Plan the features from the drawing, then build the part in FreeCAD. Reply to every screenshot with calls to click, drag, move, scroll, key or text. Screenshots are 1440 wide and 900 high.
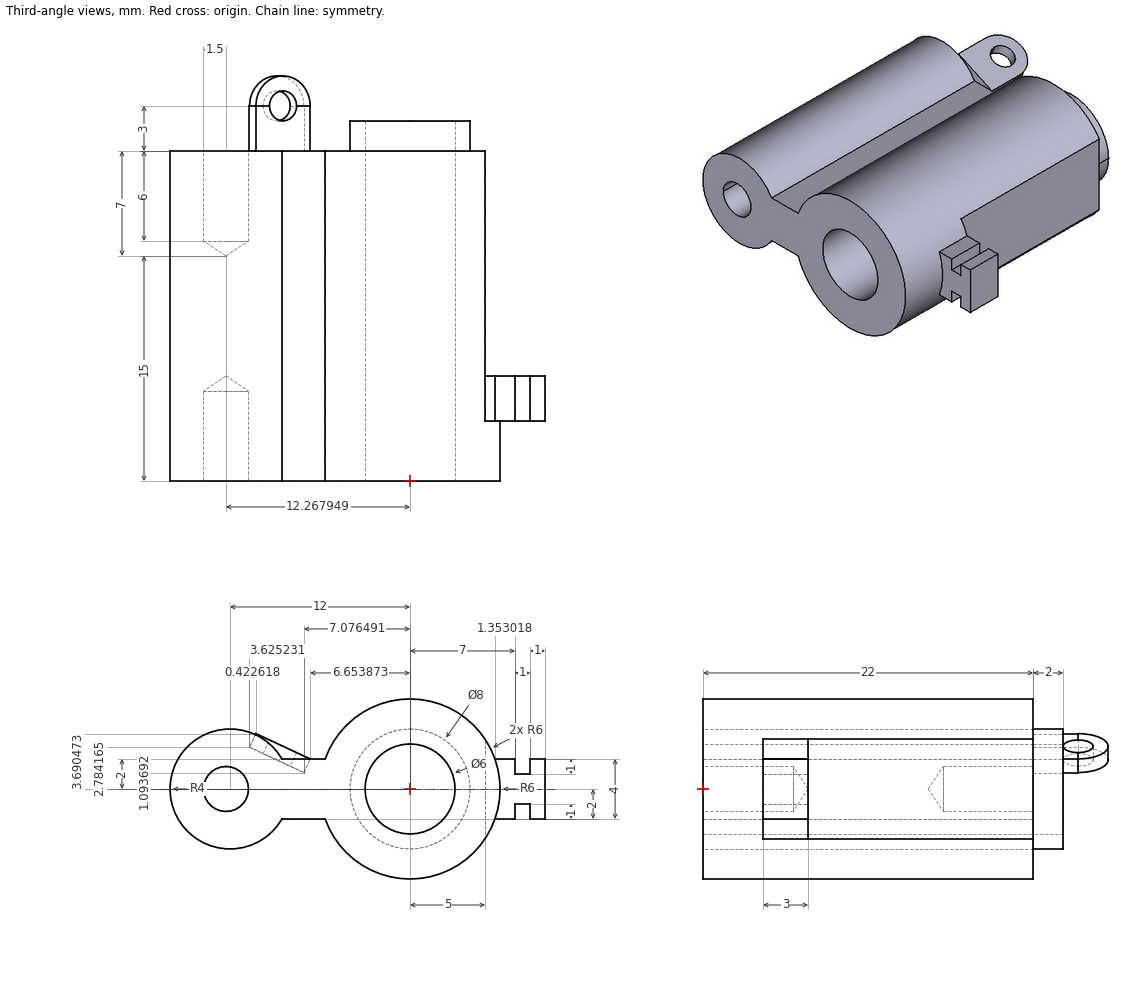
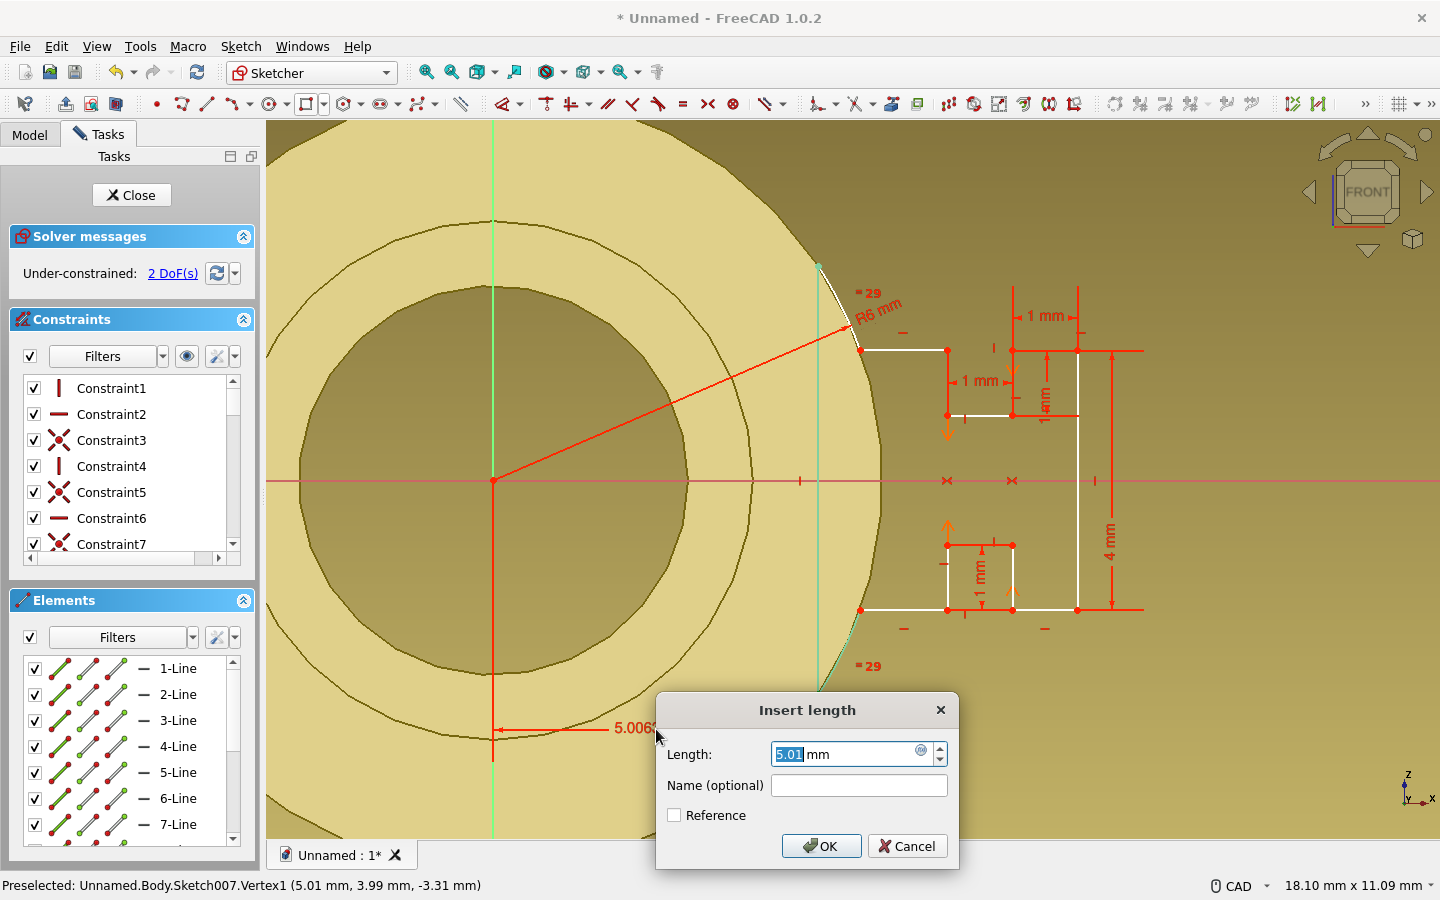
text(5)
key(Return)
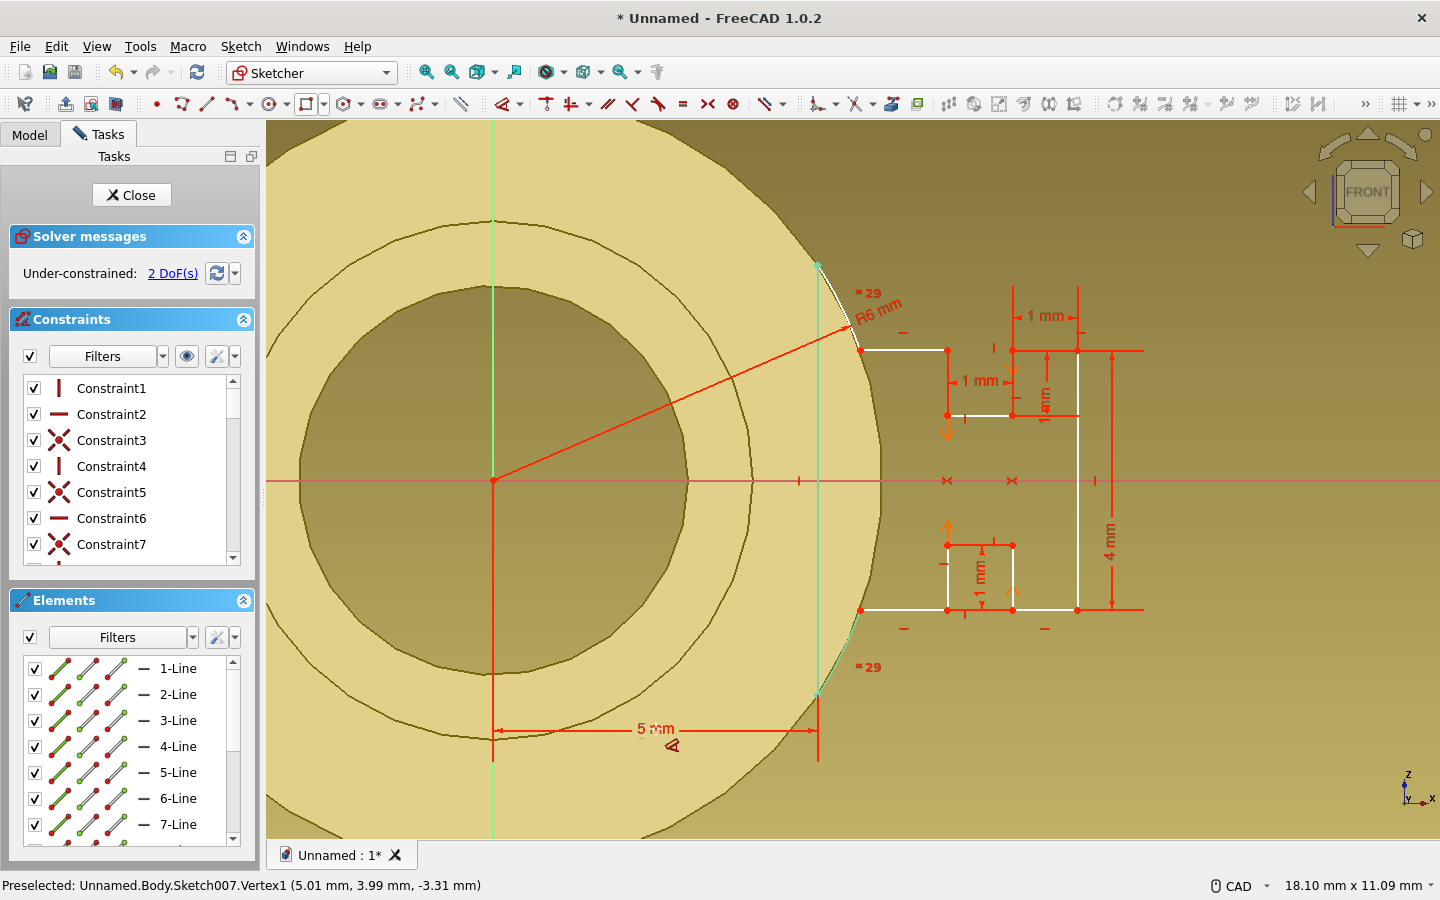
click(948, 350)
click(721, 316)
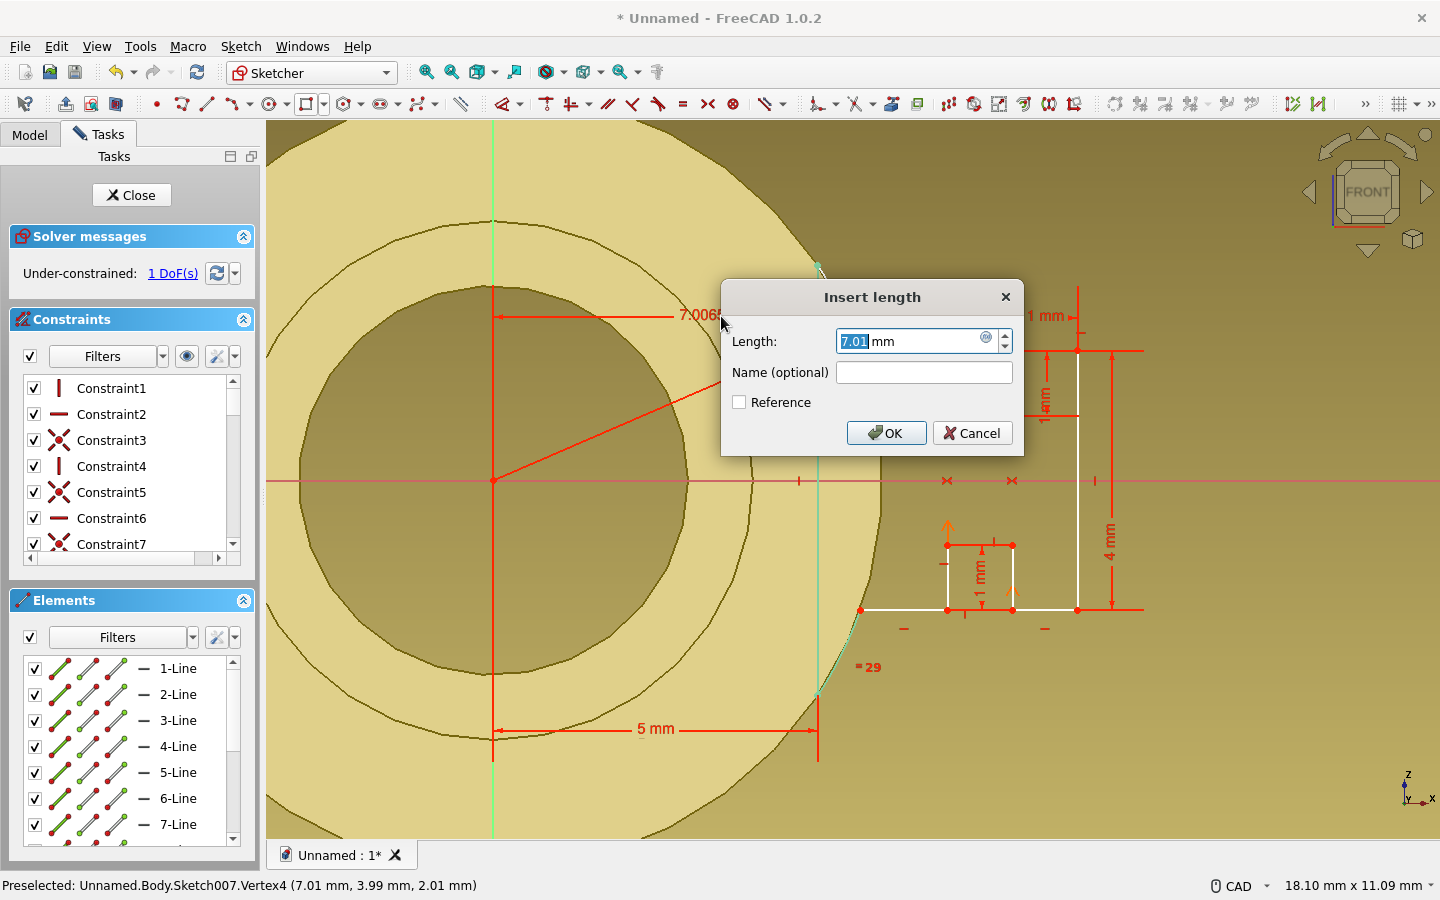
text(7)
key(Return)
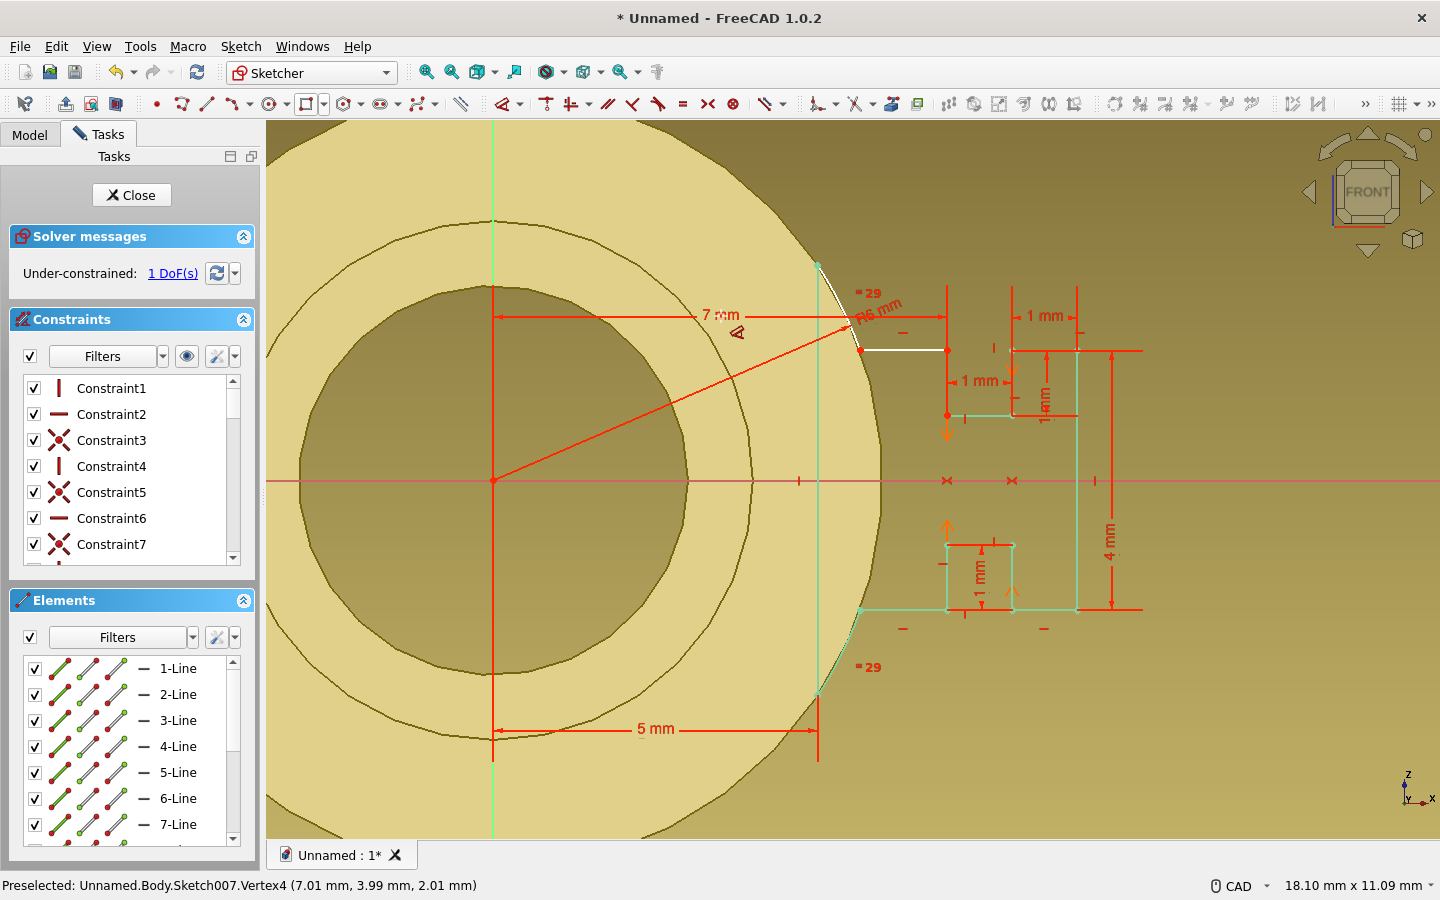
click(886, 350)
click(904, 384)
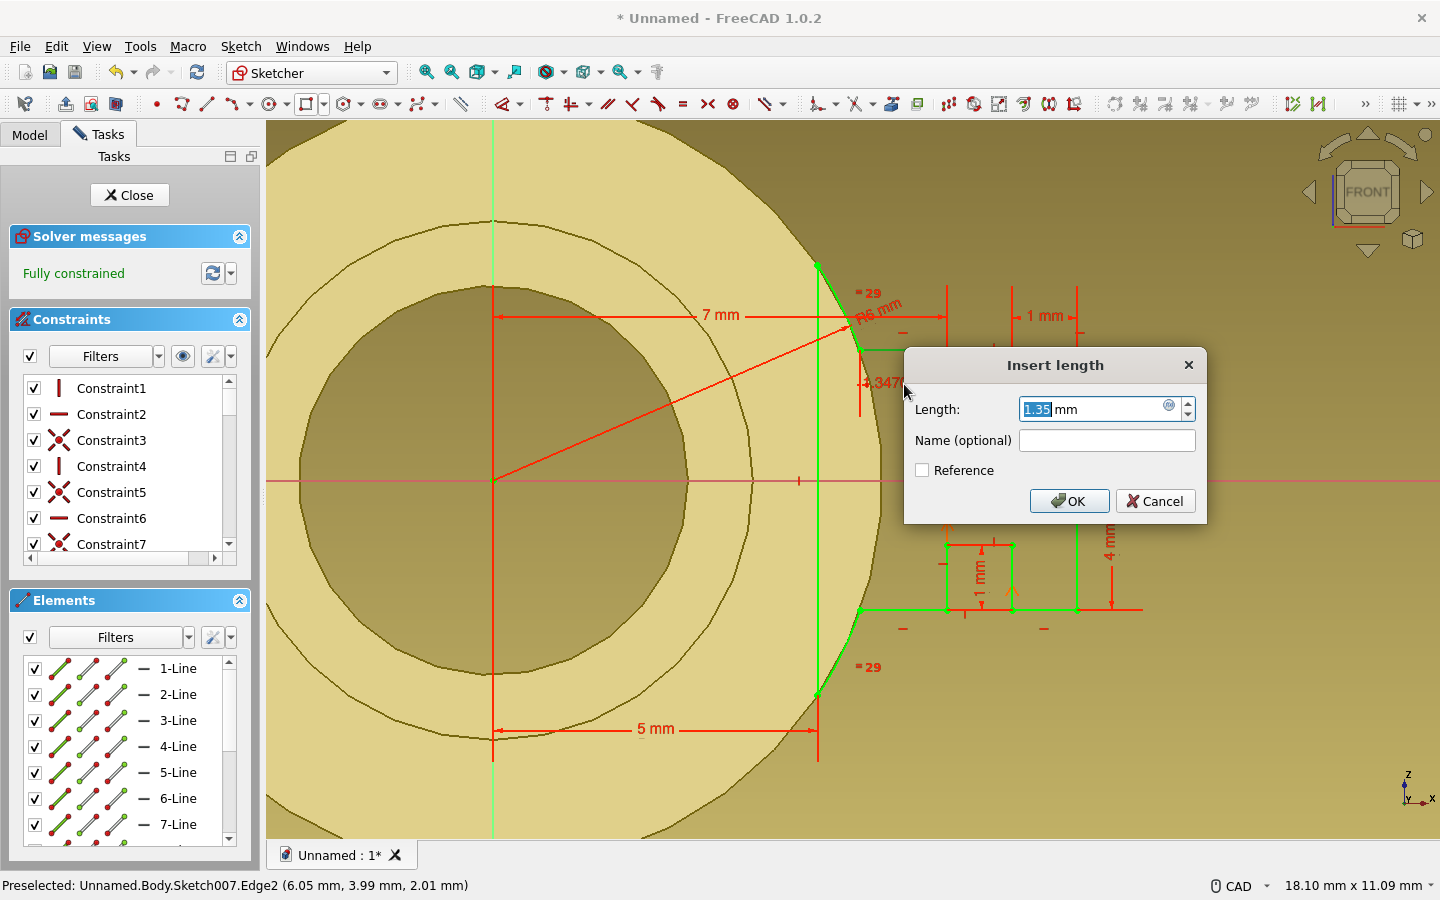
text(1.353018)
key(Return)
key(Escape)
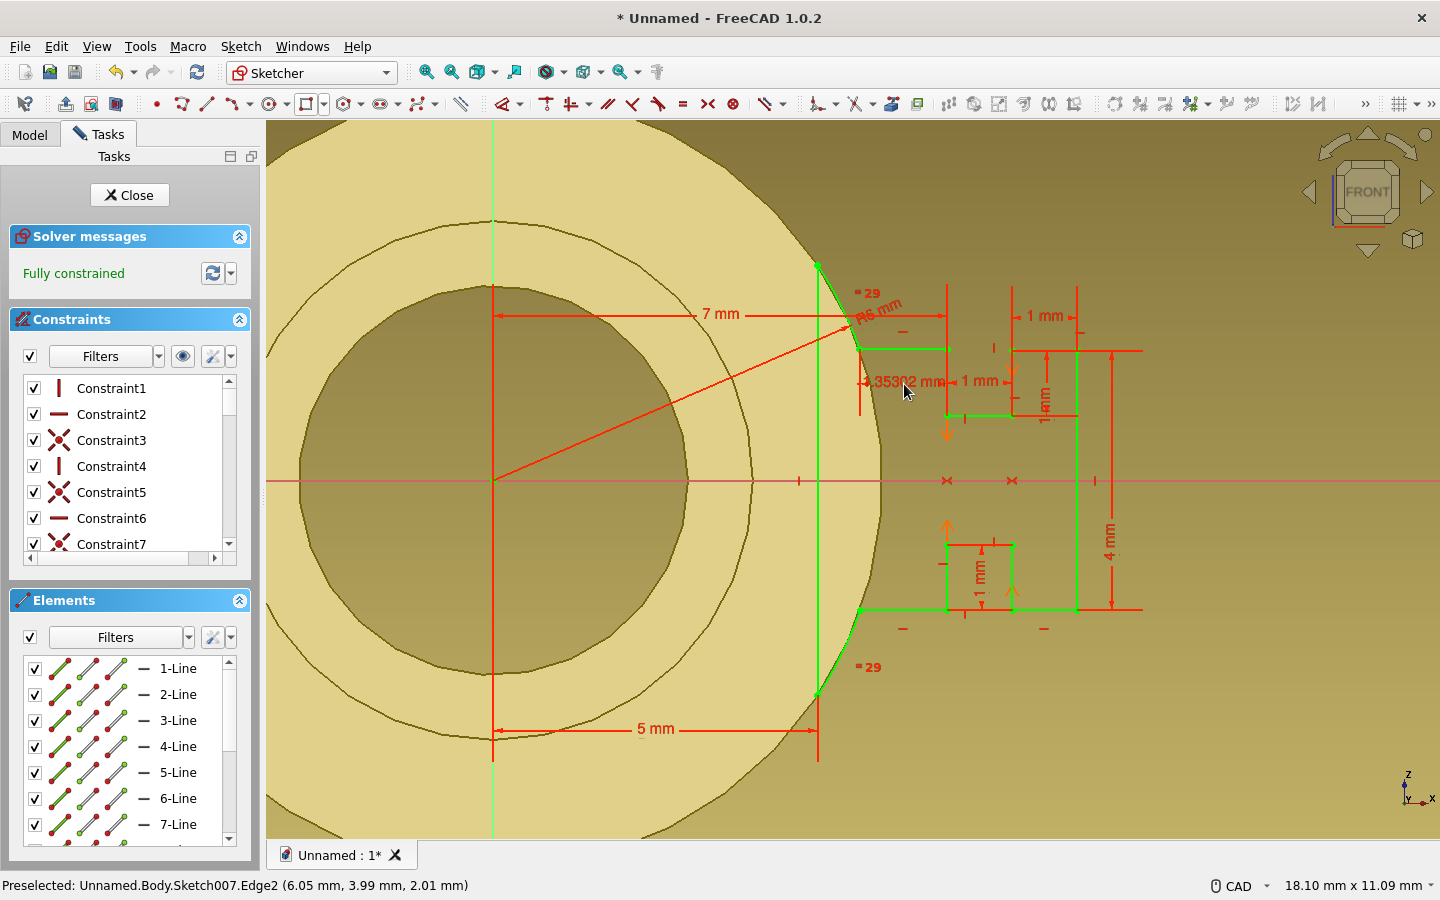
click(130, 195)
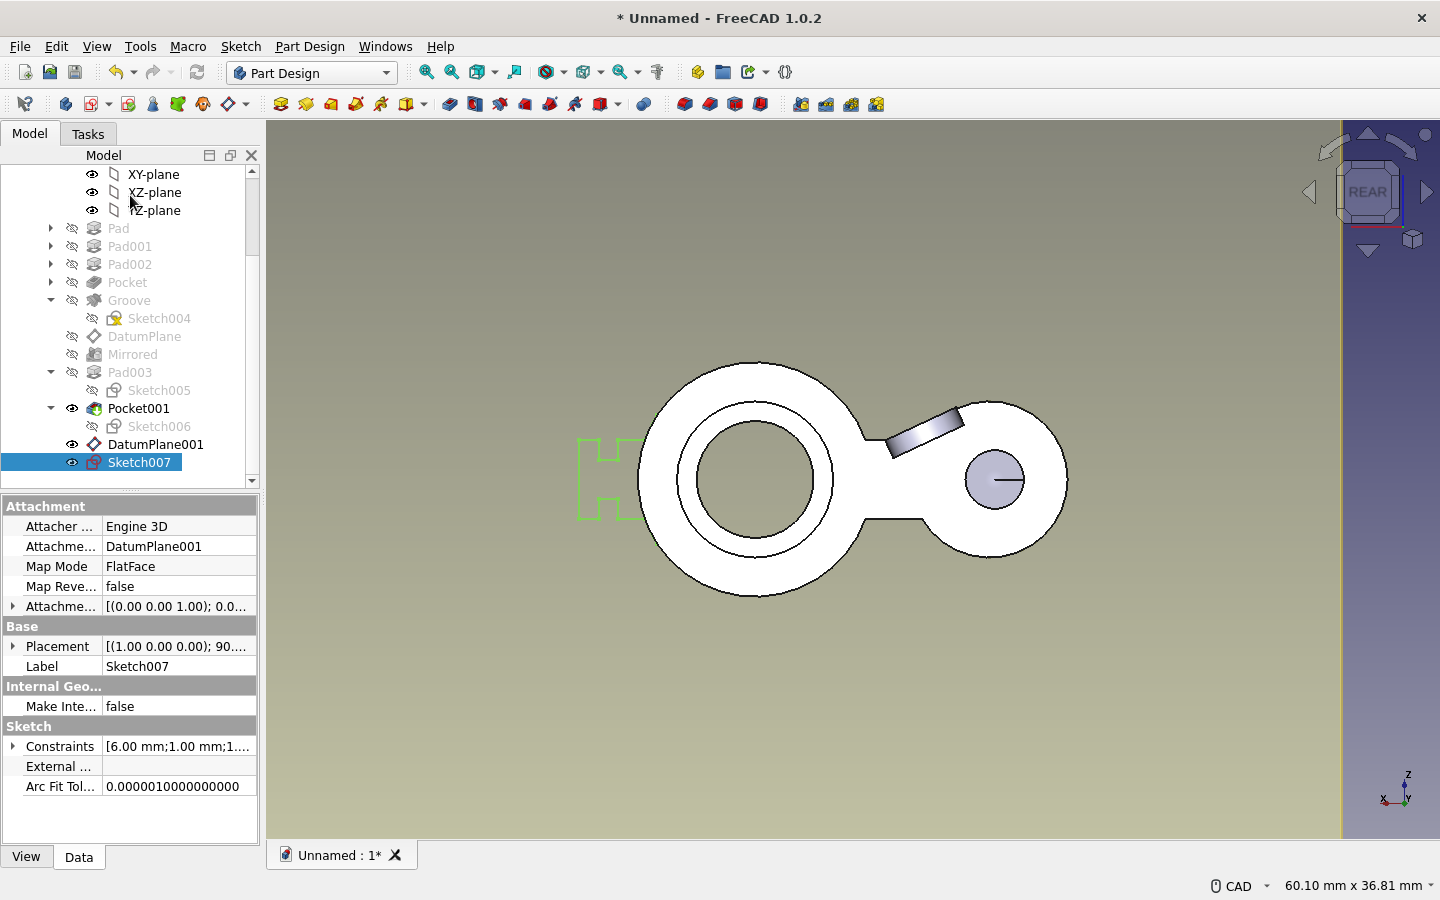
click(281, 104)